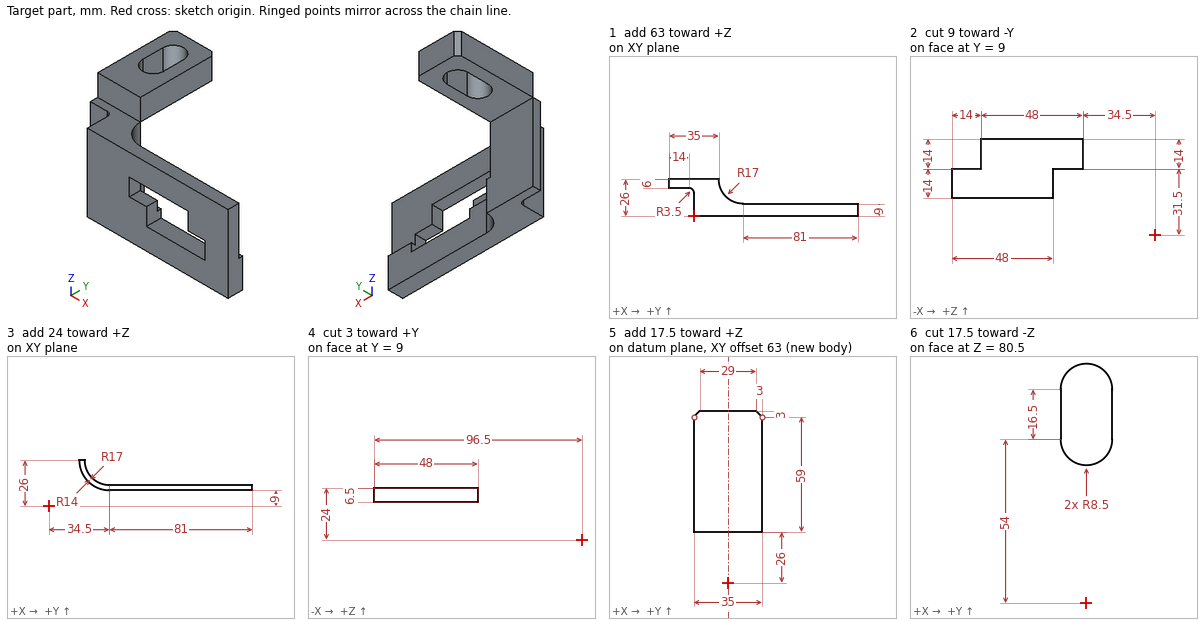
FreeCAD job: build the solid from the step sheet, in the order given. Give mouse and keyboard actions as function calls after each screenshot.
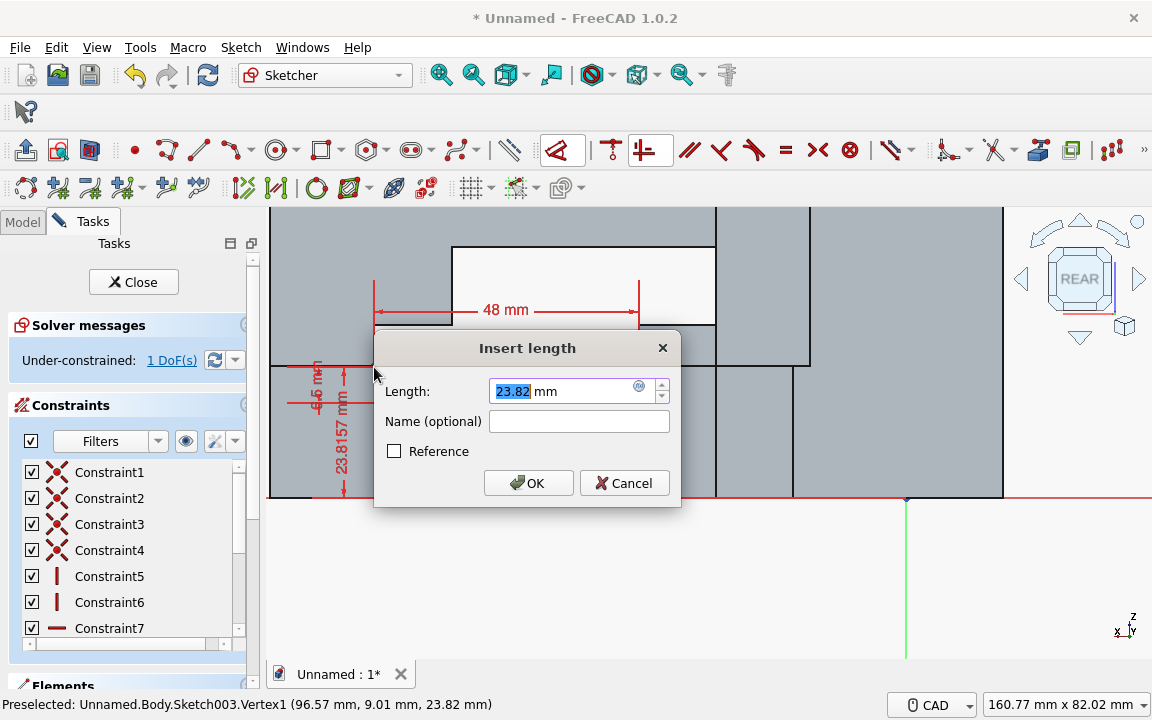
text(24)
key(Return)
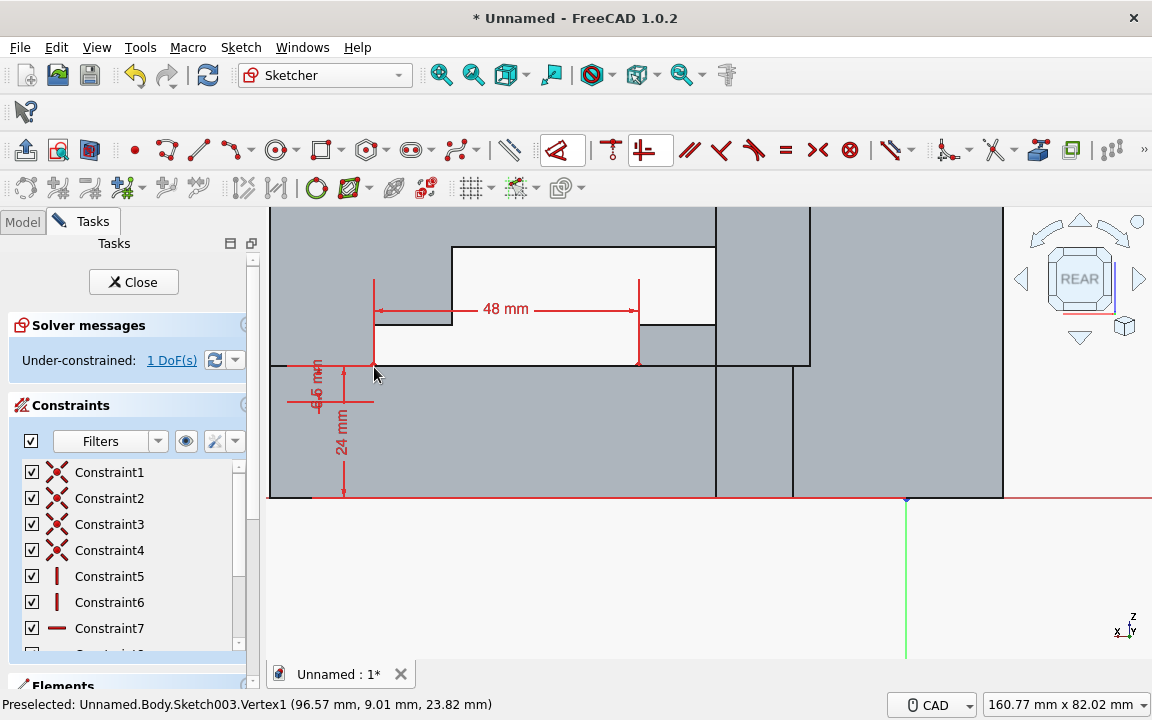
click(374, 366)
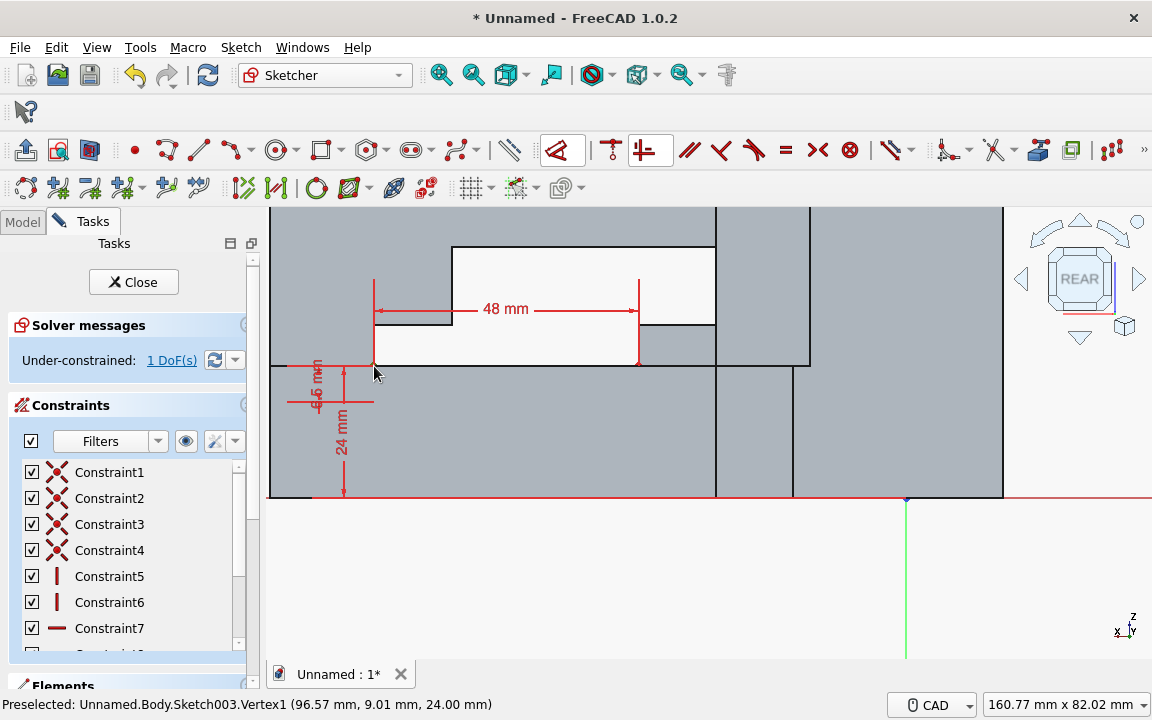
key(l)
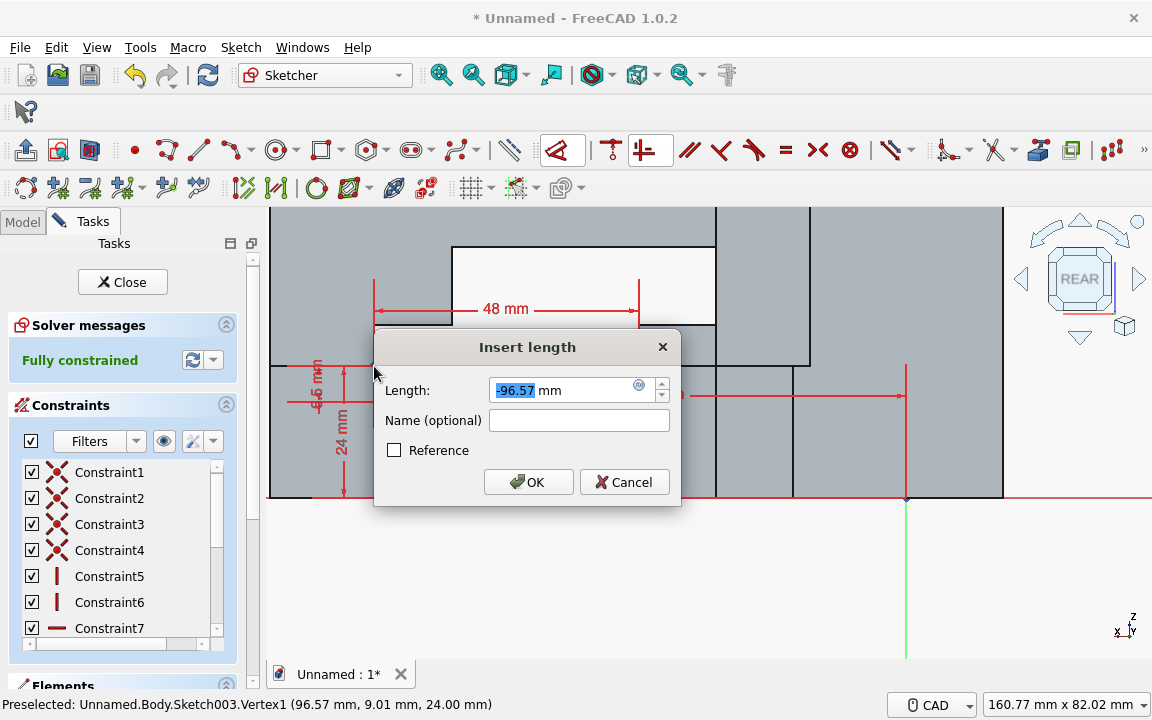
text(-96.5)
key(Return)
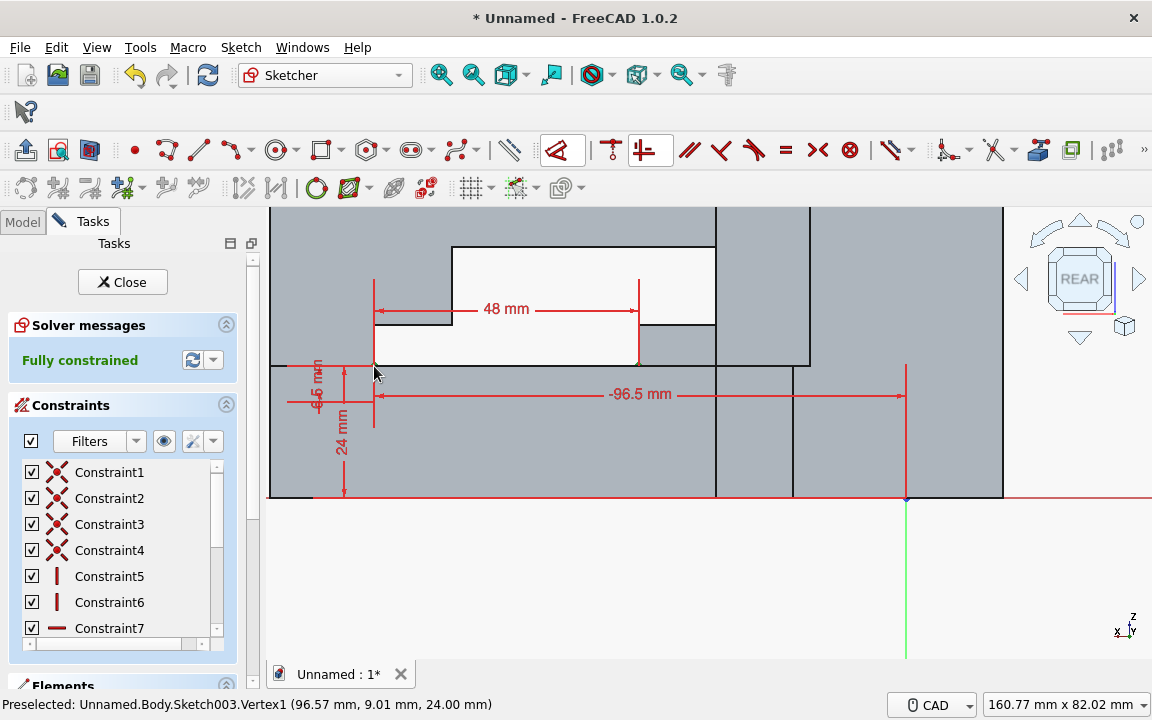
click(123, 282)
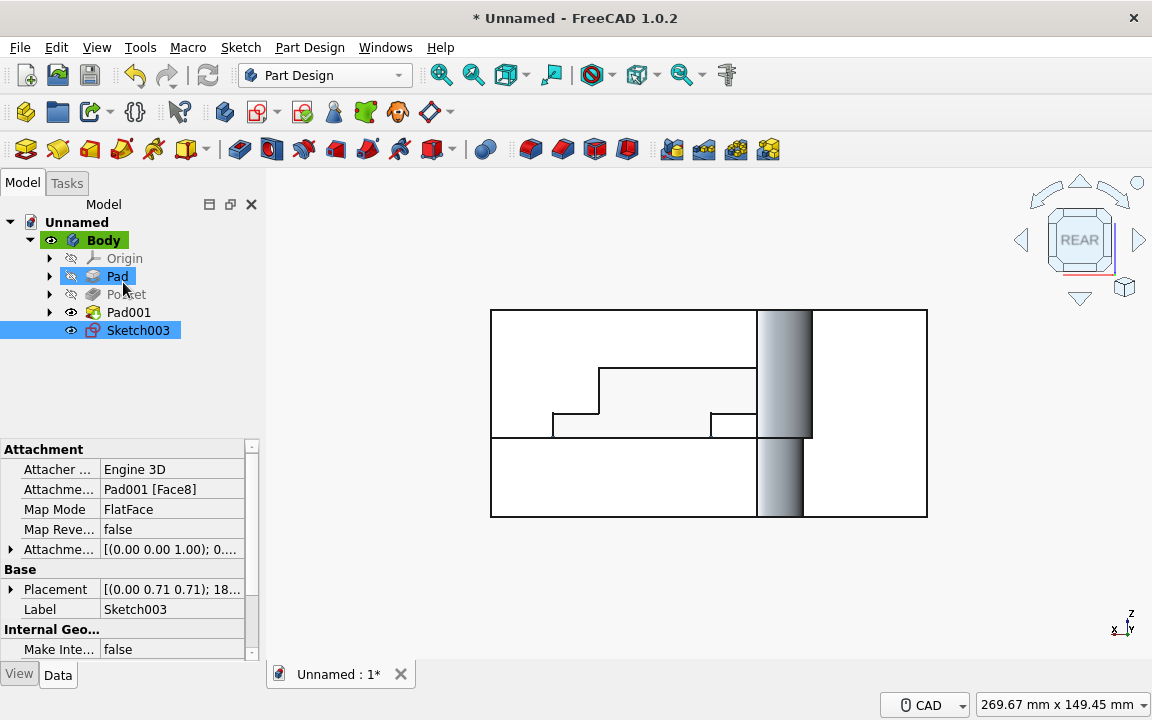
click(240, 150)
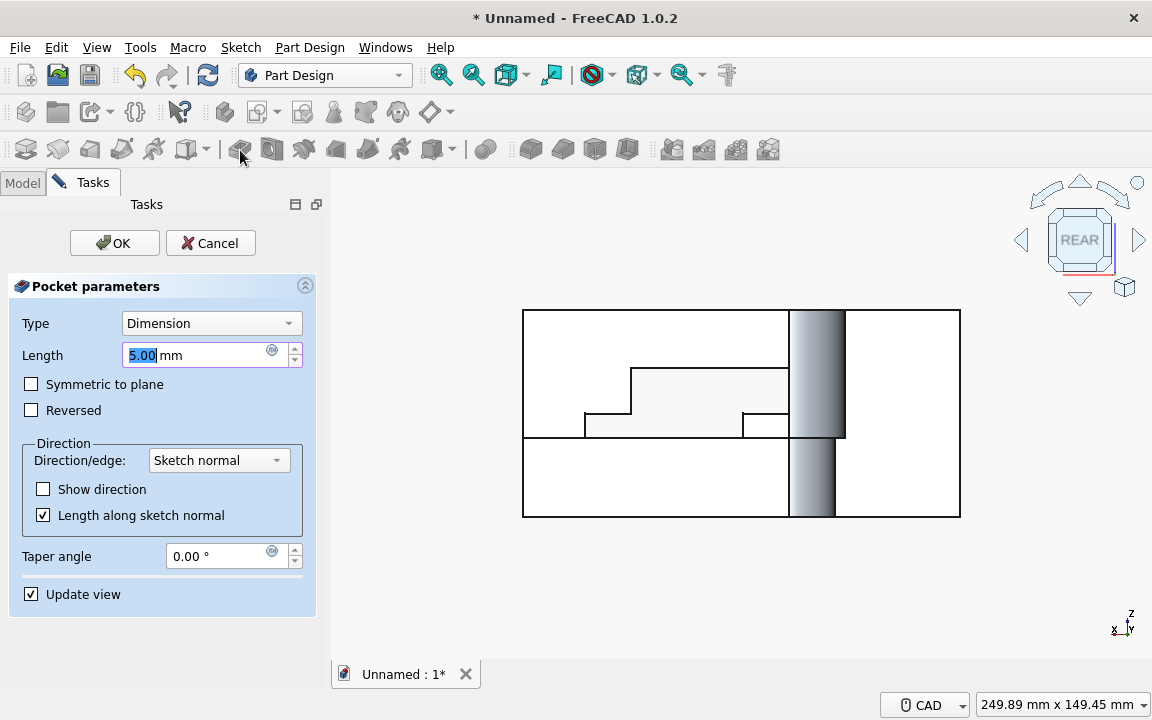
text(3)
key(Tab)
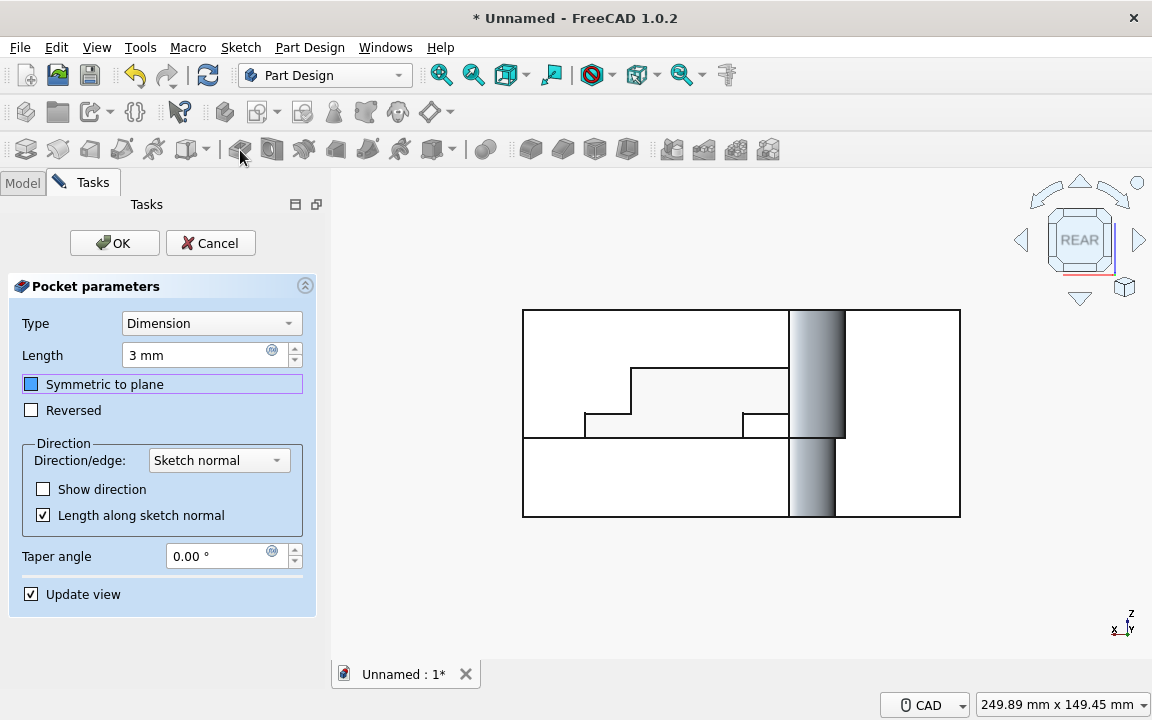
click(30, 410)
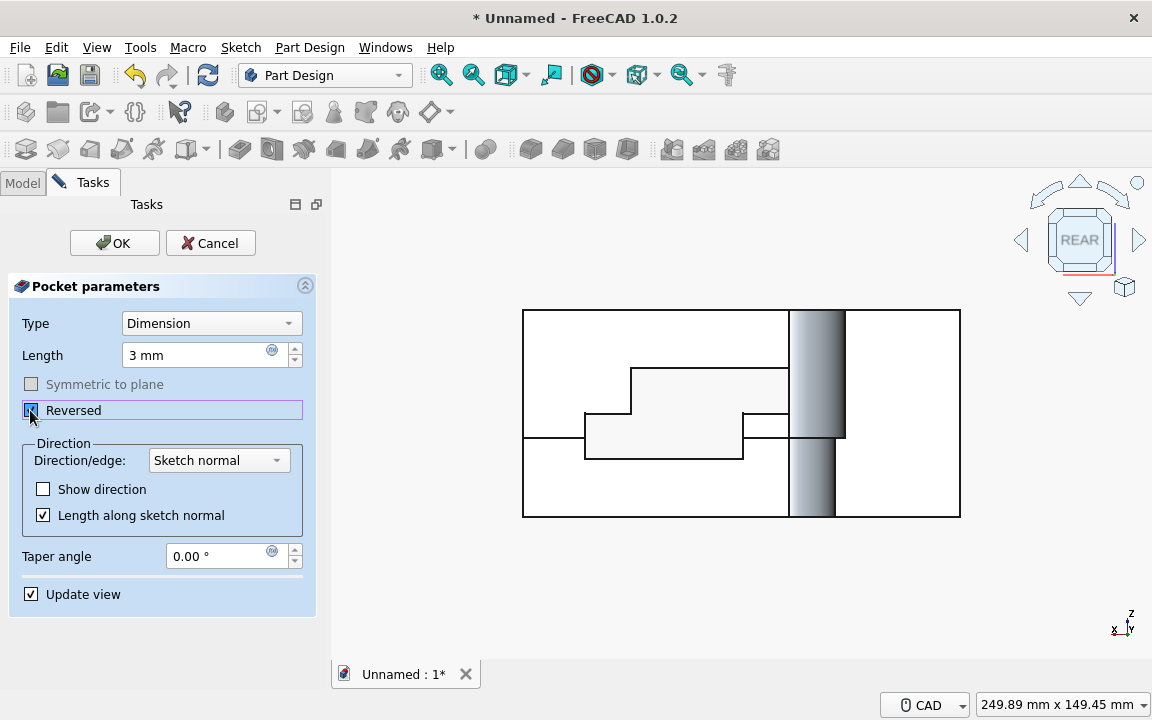
click(115, 243)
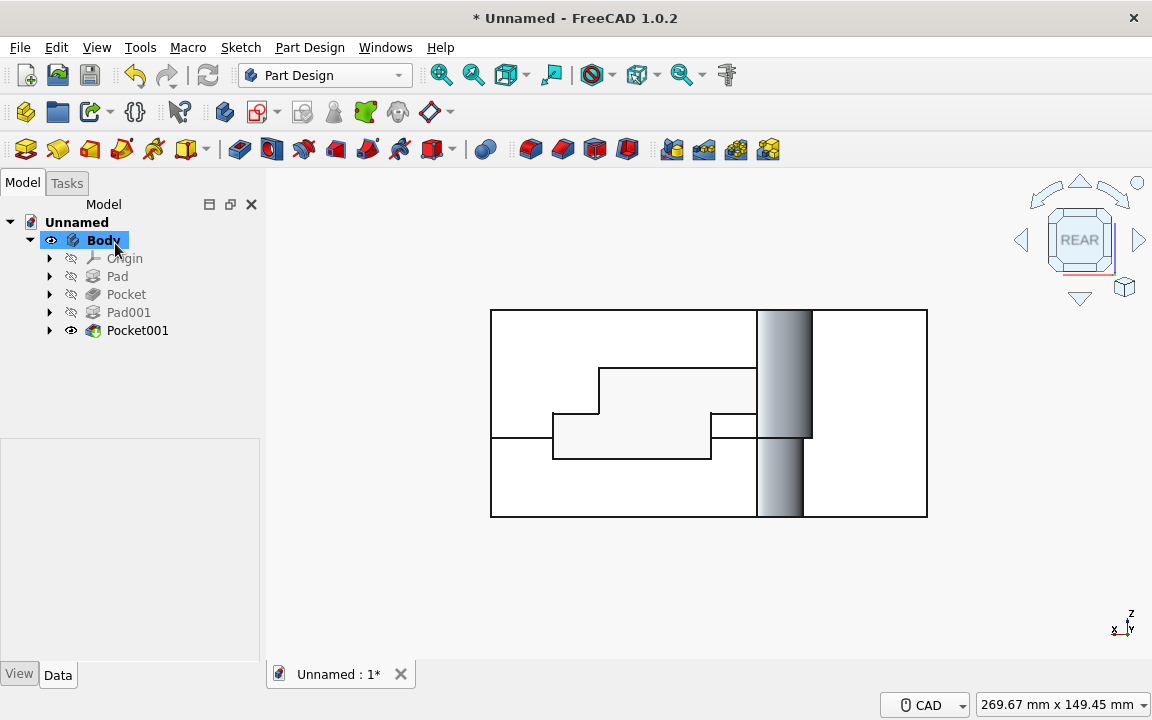
click(226, 112)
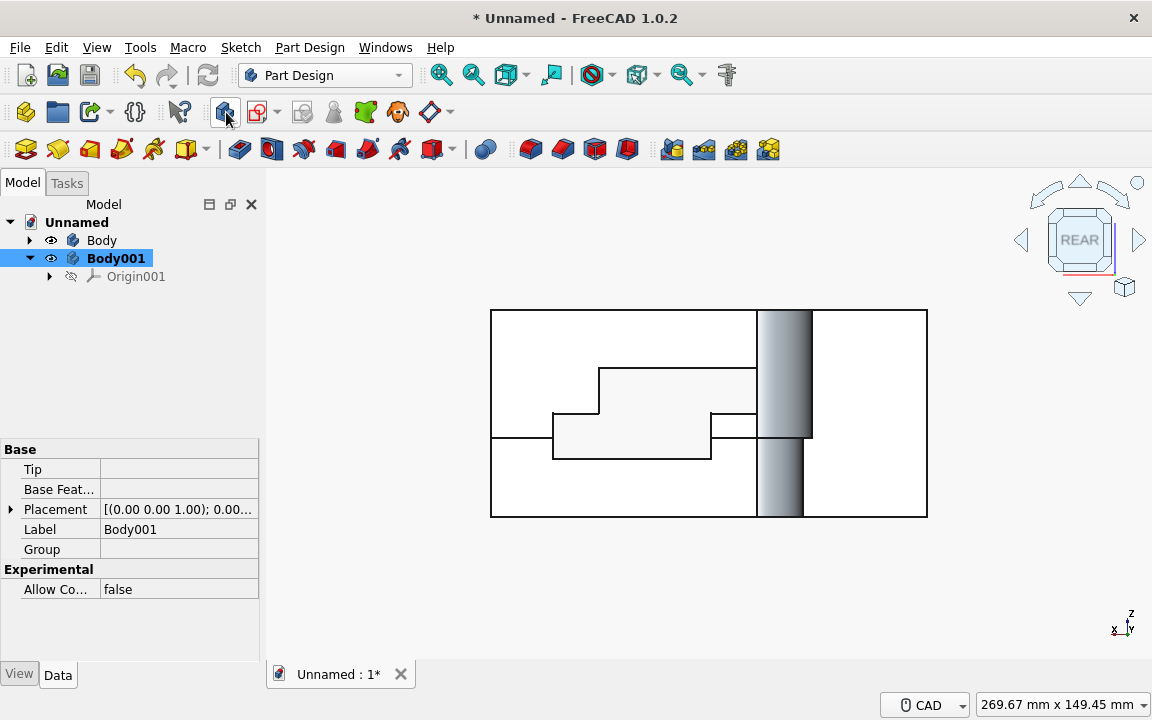
click(50, 276)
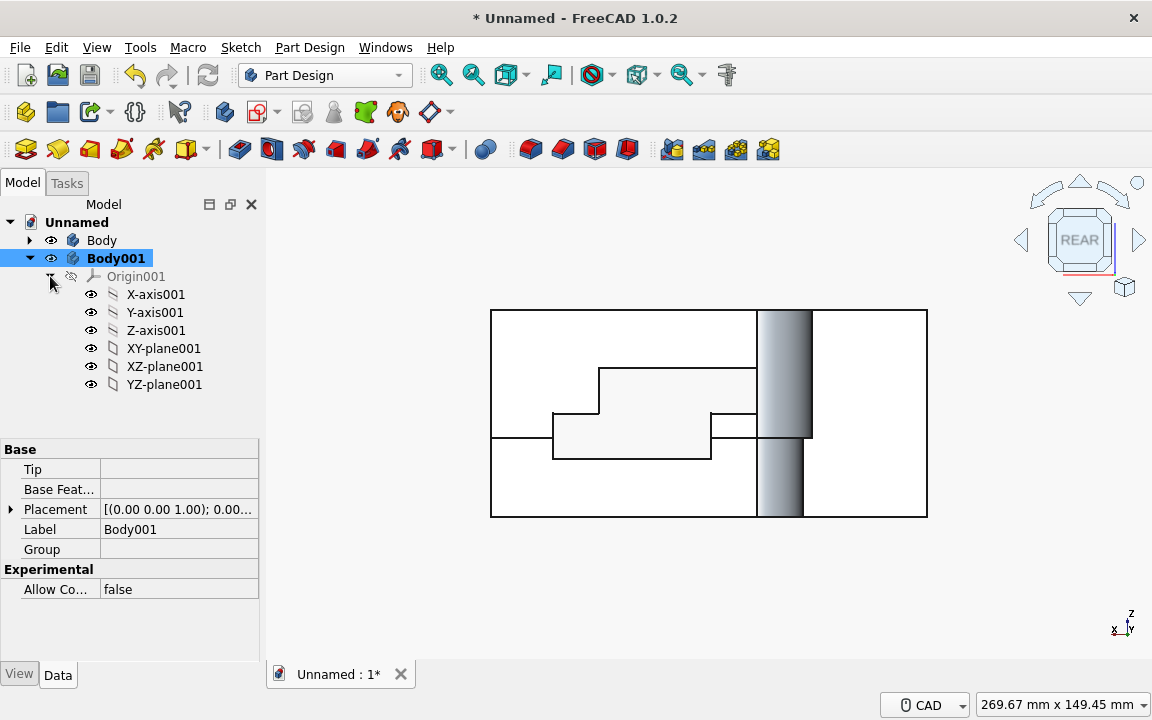
click(136, 348)